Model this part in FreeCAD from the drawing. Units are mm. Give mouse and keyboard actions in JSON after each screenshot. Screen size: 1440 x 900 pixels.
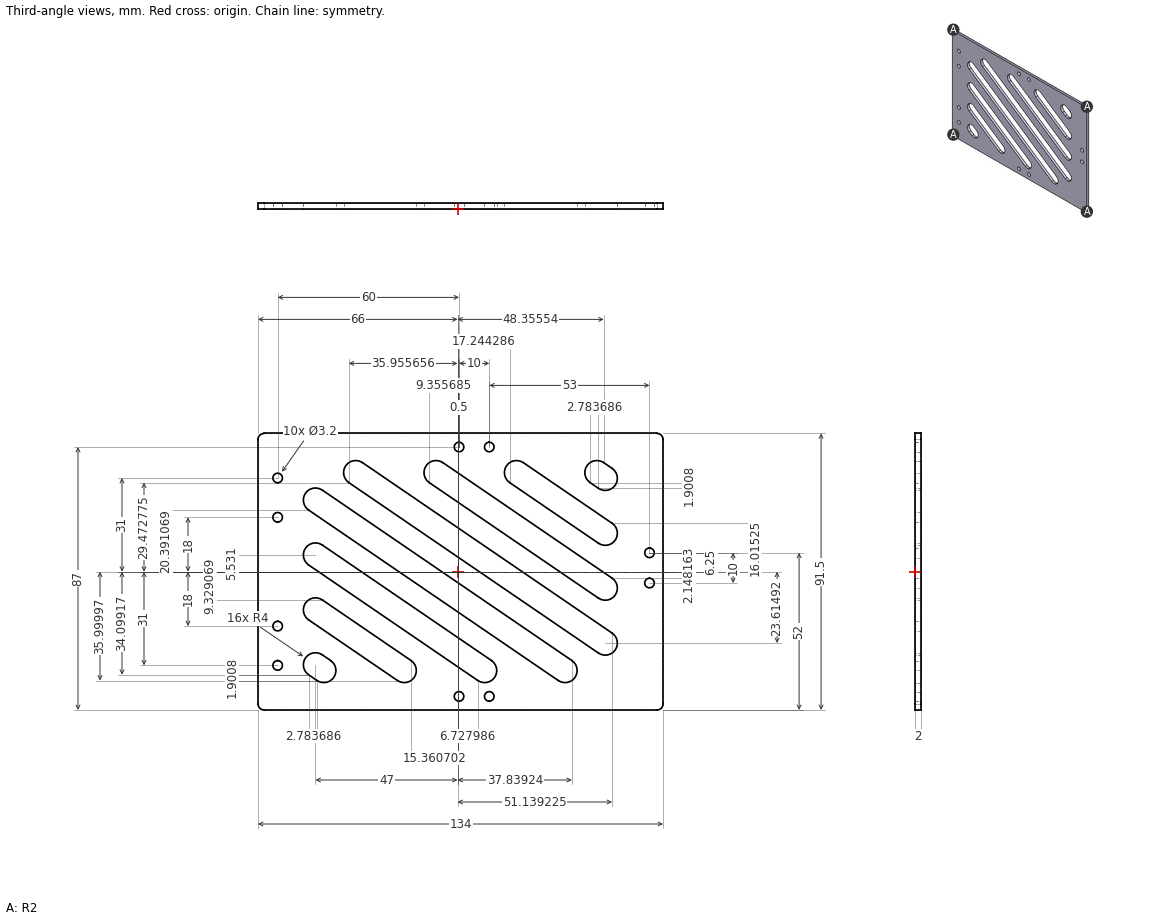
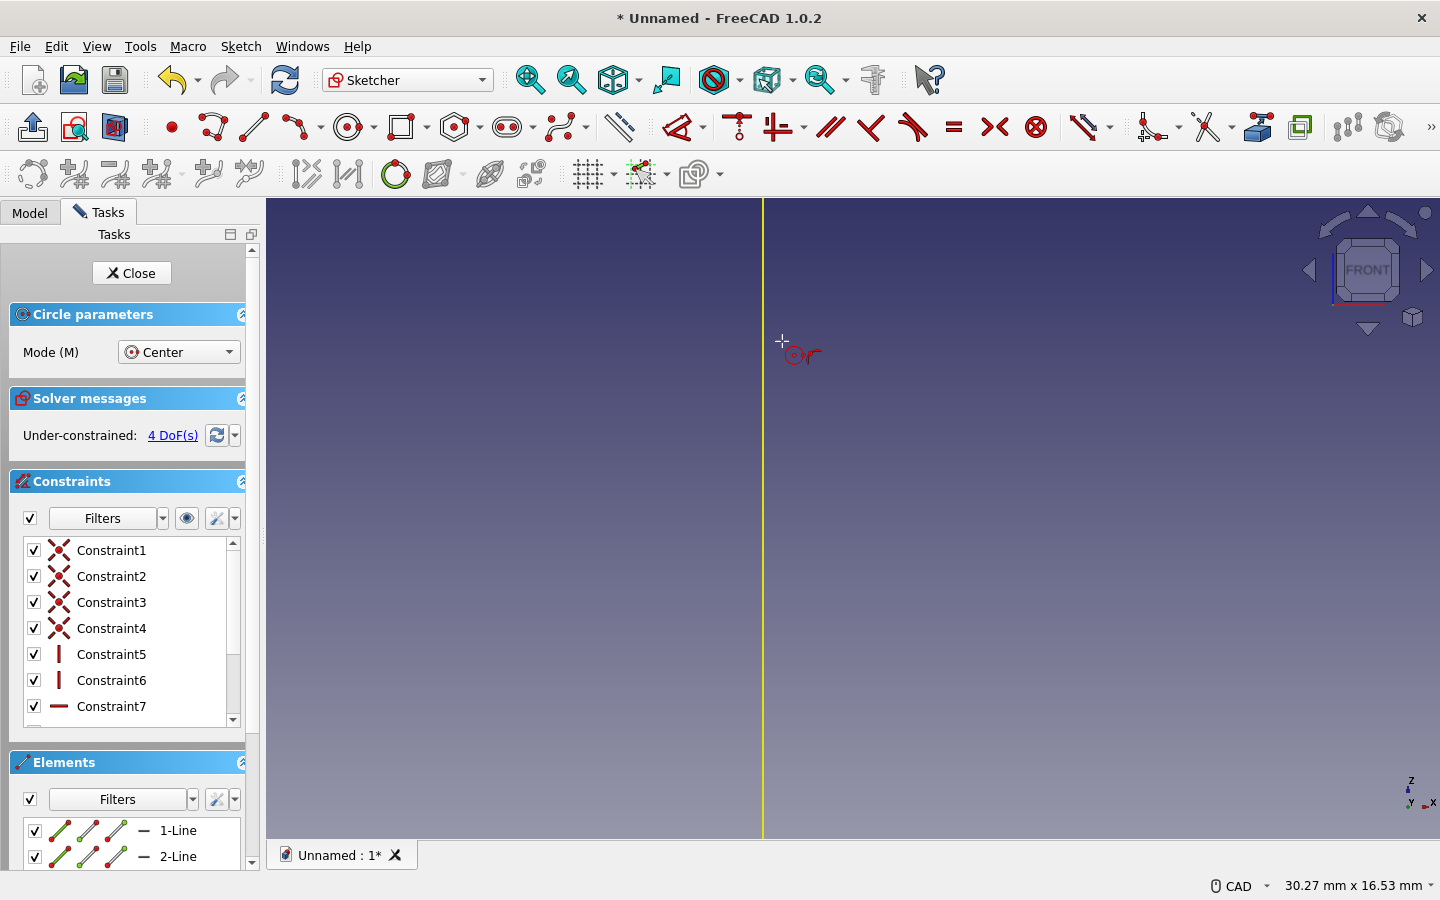
{"action": "left_click", "coordinate": [782, 342]}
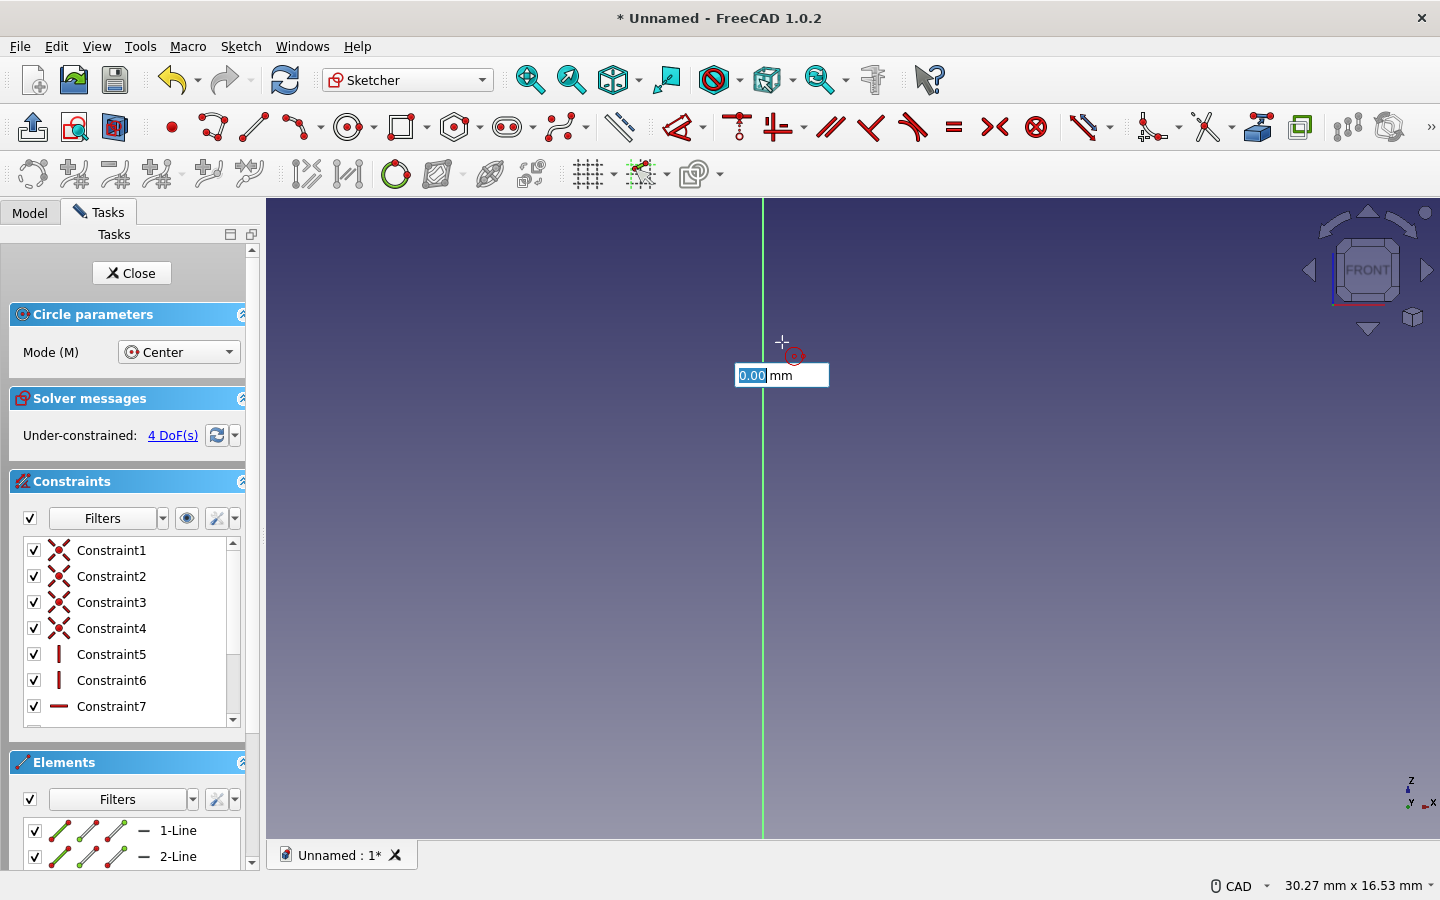
{"action": "scroll", "coordinate": [782, 341], "scroll_direction": "down", "scroll_amount": 11}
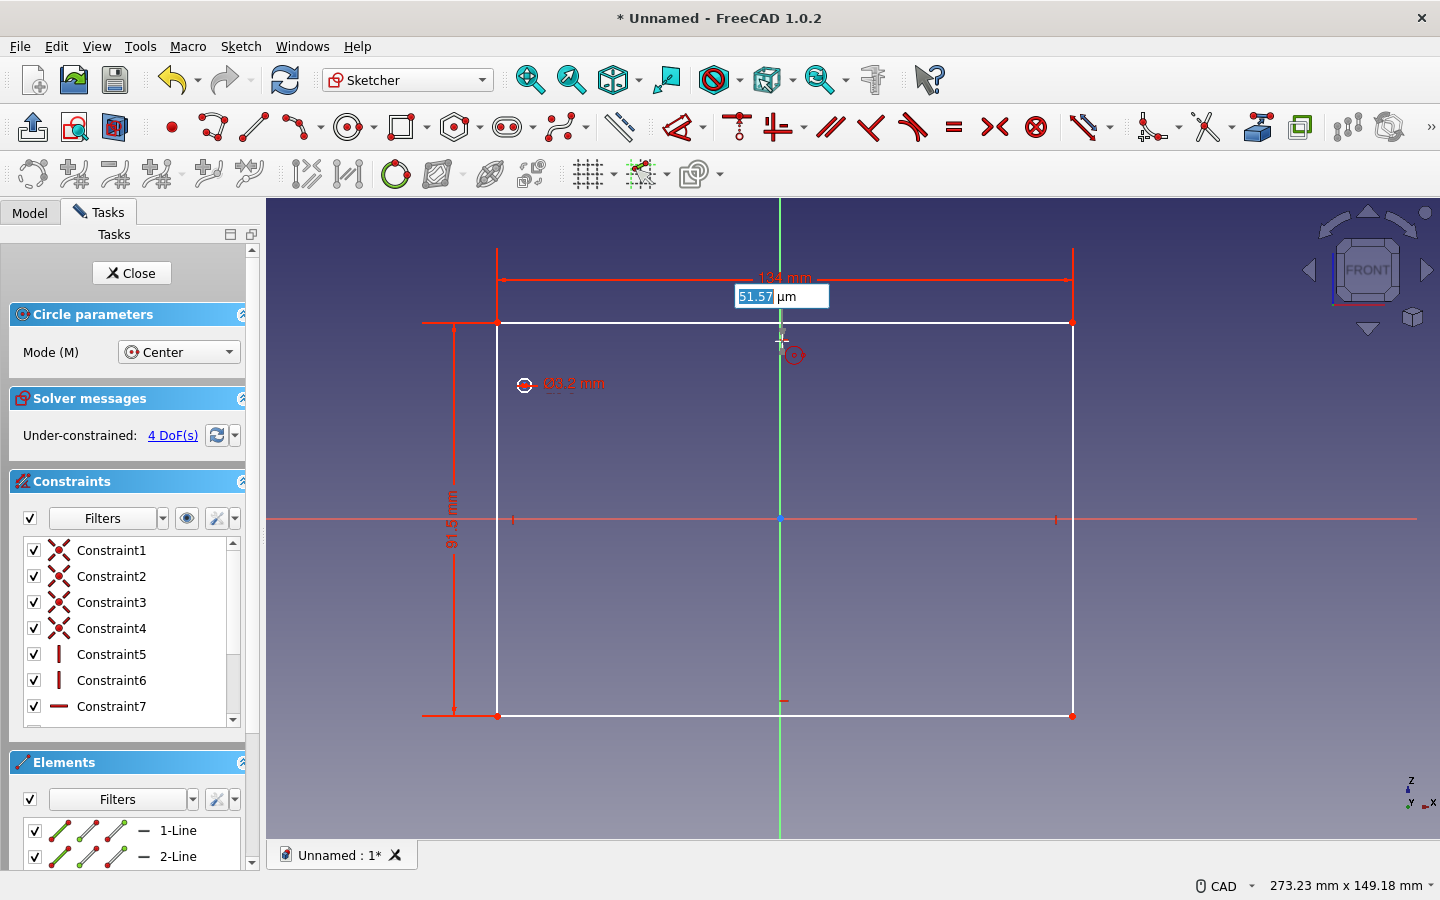
{"action": "scroll", "coordinate": [787, 336], "scroll_direction": "up", "scroll_amount": 5}
{"action": "mouse_move", "coordinate": [787, 337]}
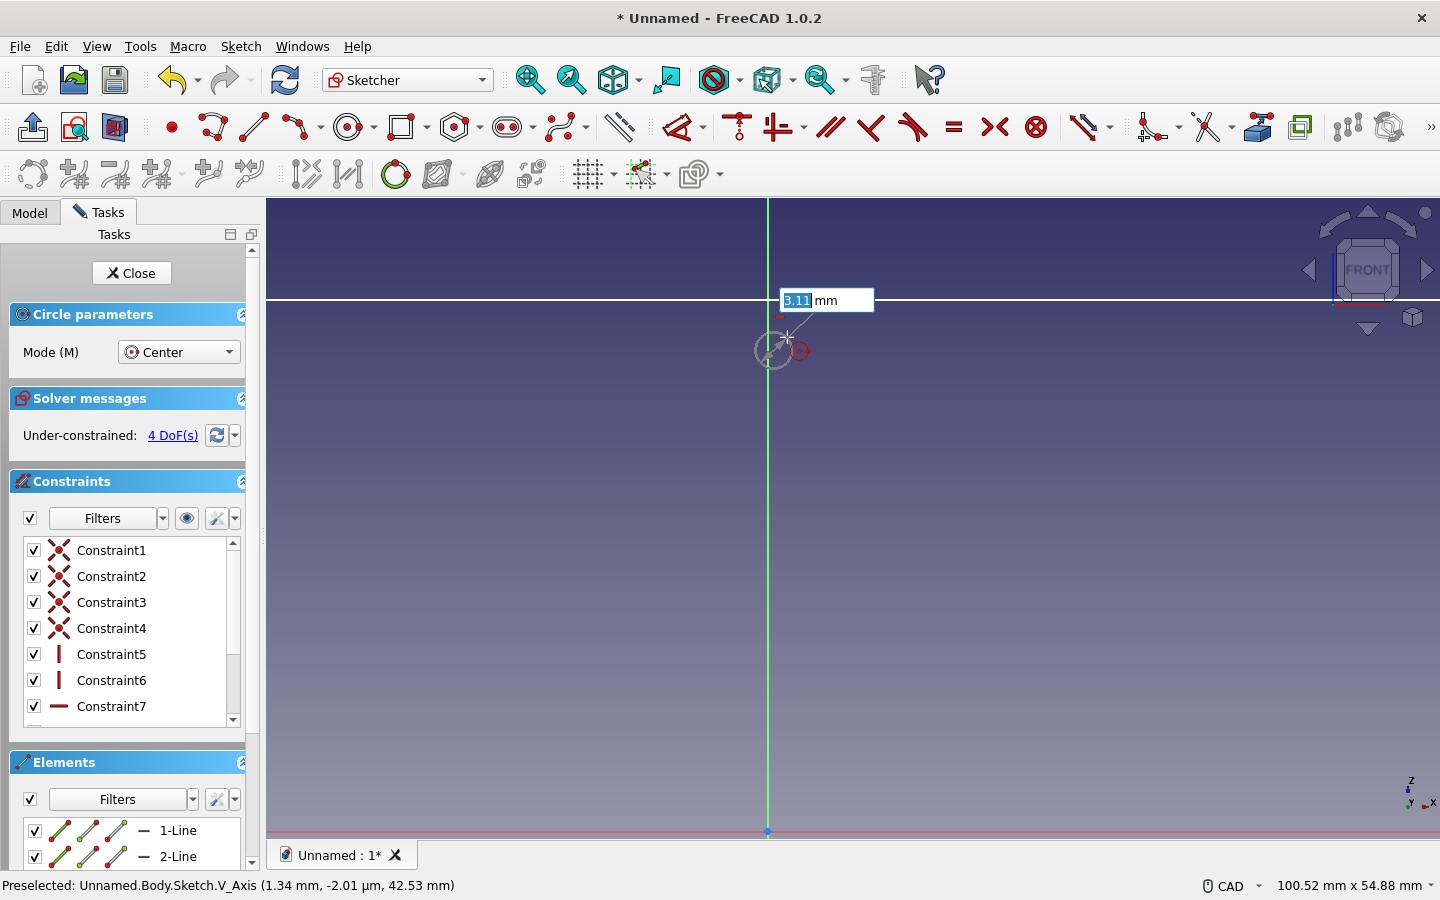
{"action": "type", "text": "3.2"}
{"action": "key", "text": "Return"}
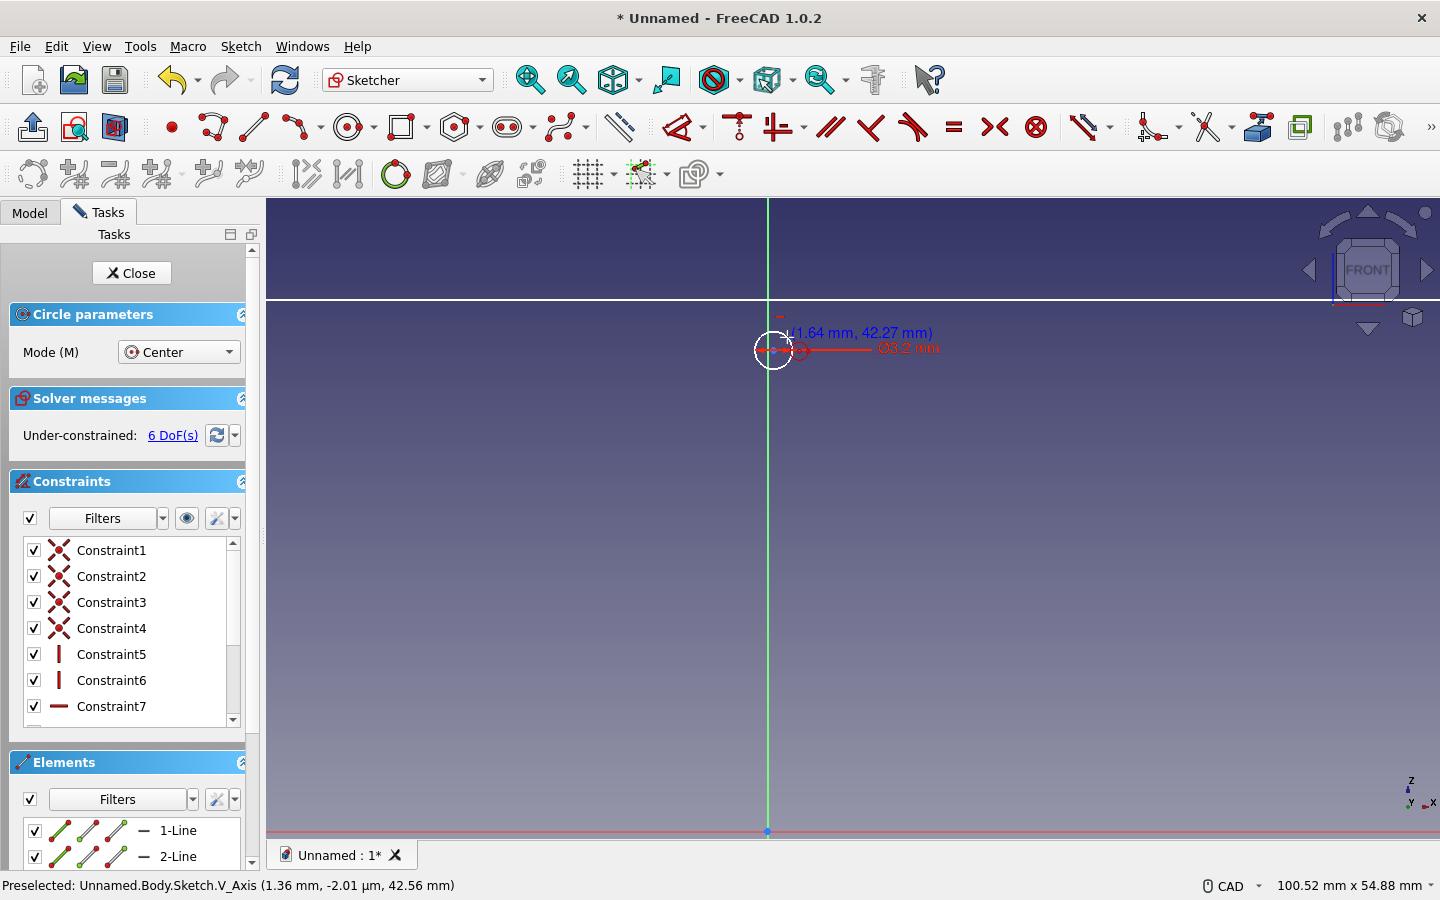
{"action": "scroll", "coordinate": [787, 336], "scroll_direction": "down", "scroll_amount": 5}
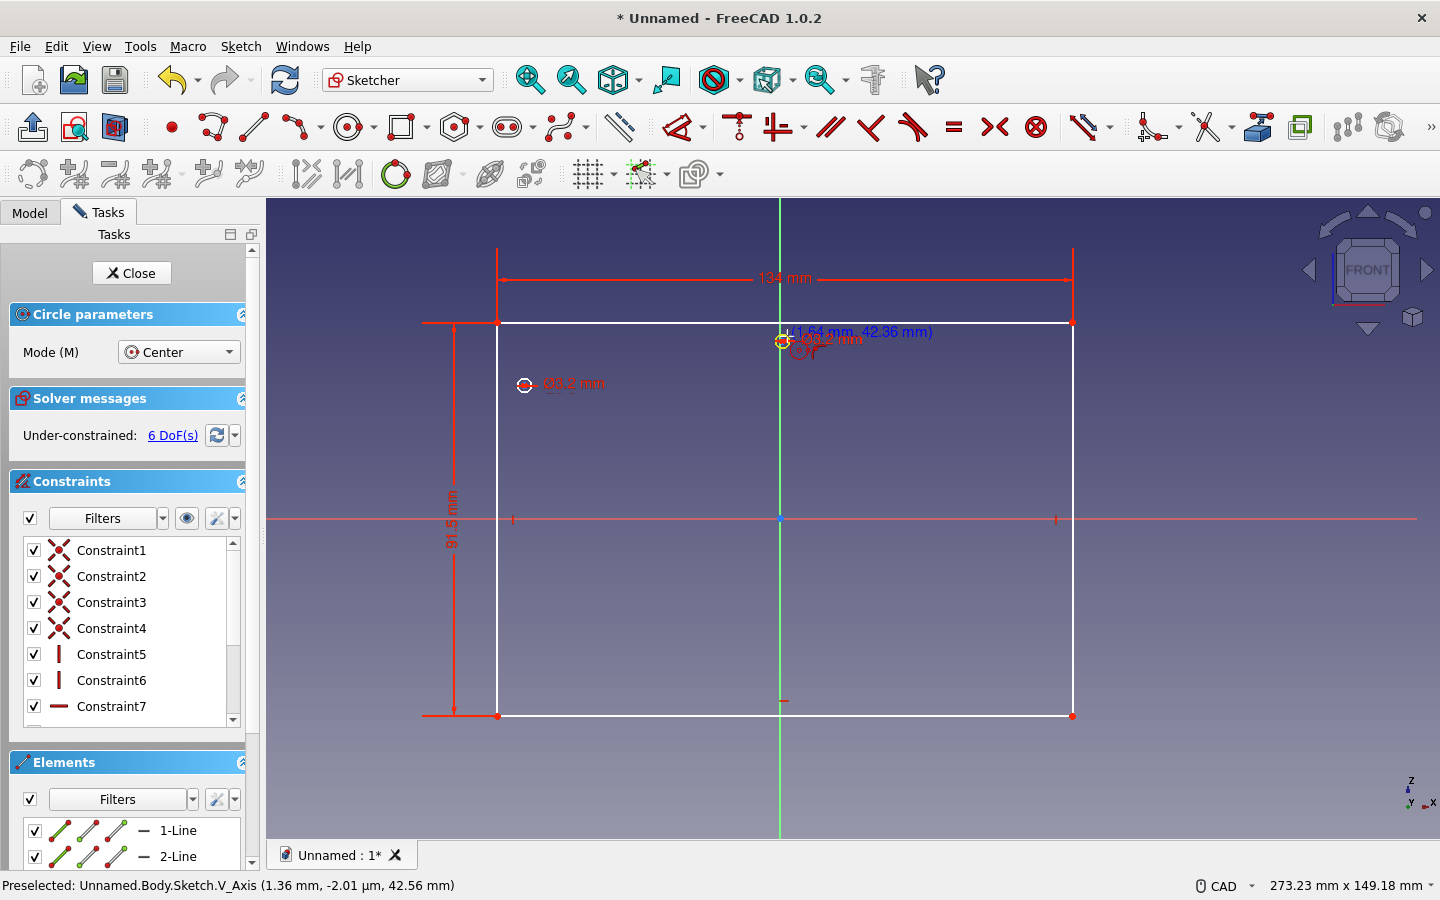
{"action": "scroll", "coordinate": [525, 441], "scroll_direction": "up", "scroll_amount": 6}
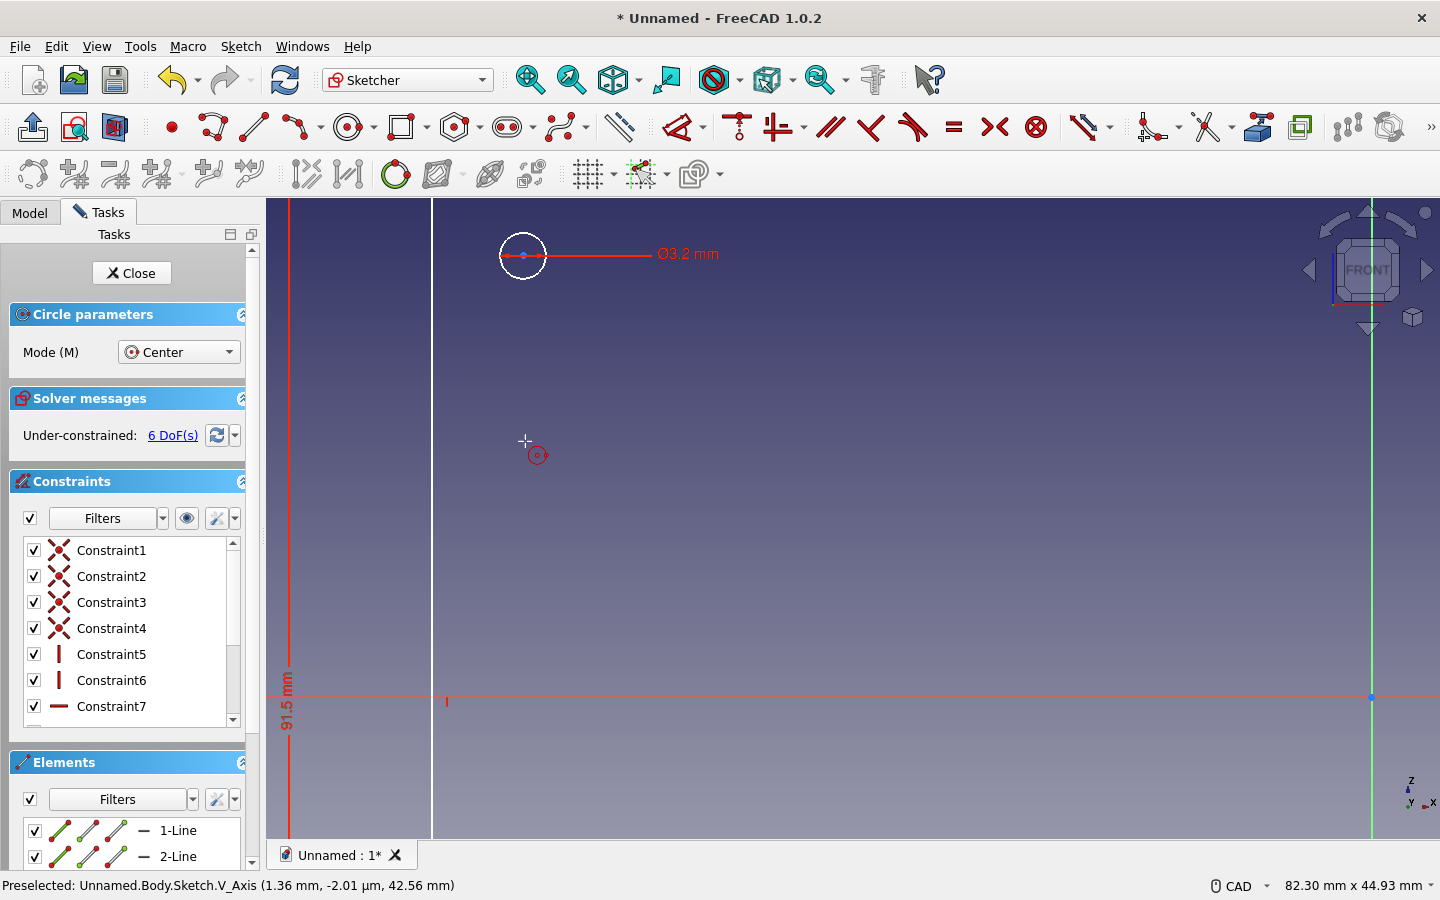
{"action": "left_click", "coordinate": [523, 441]}
{"action": "mouse_move", "coordinate": [539, 425]}